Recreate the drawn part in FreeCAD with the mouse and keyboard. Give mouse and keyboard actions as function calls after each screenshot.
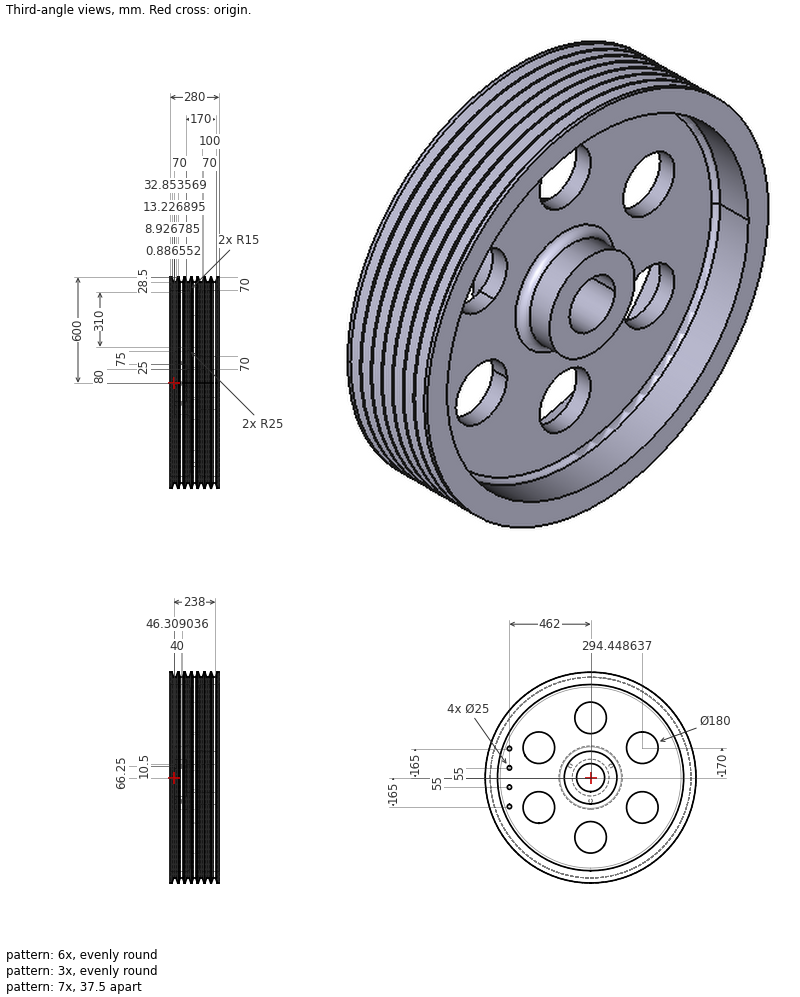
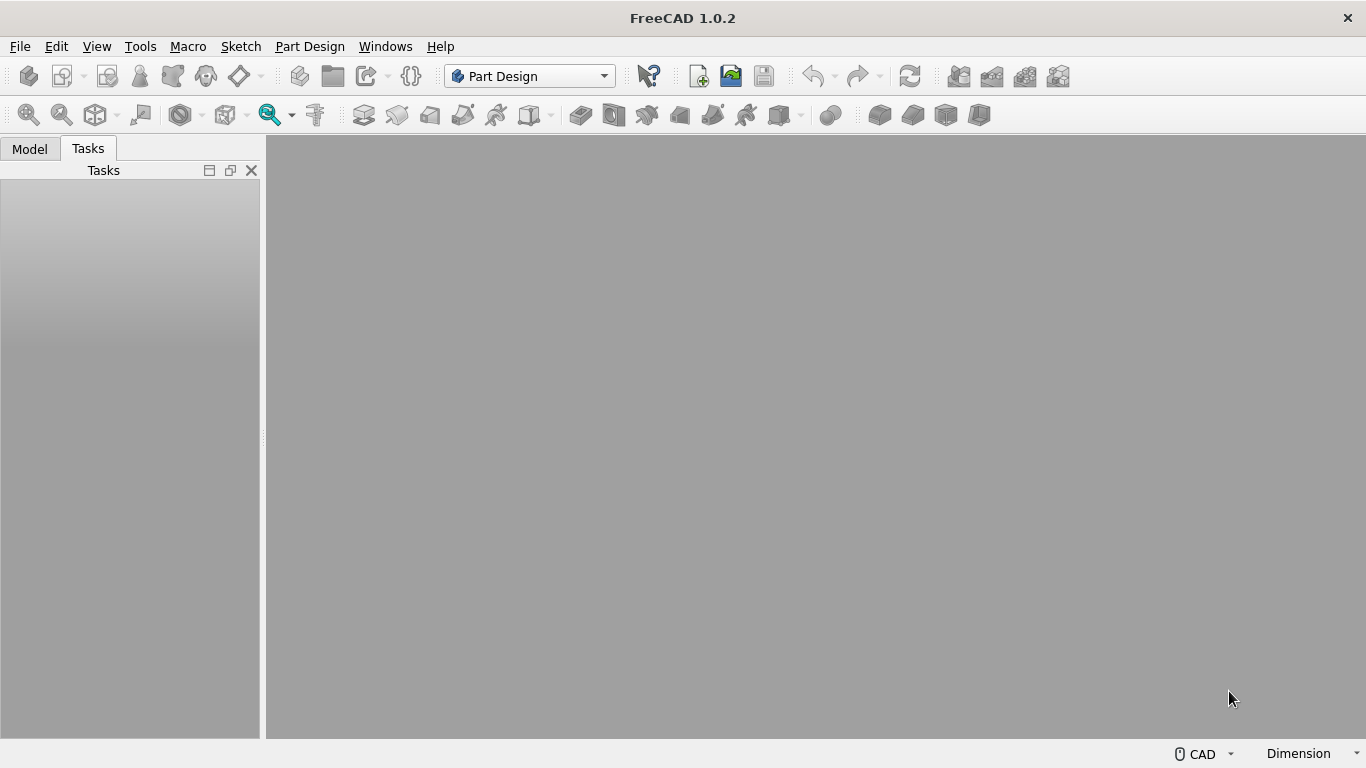
click(698, 76)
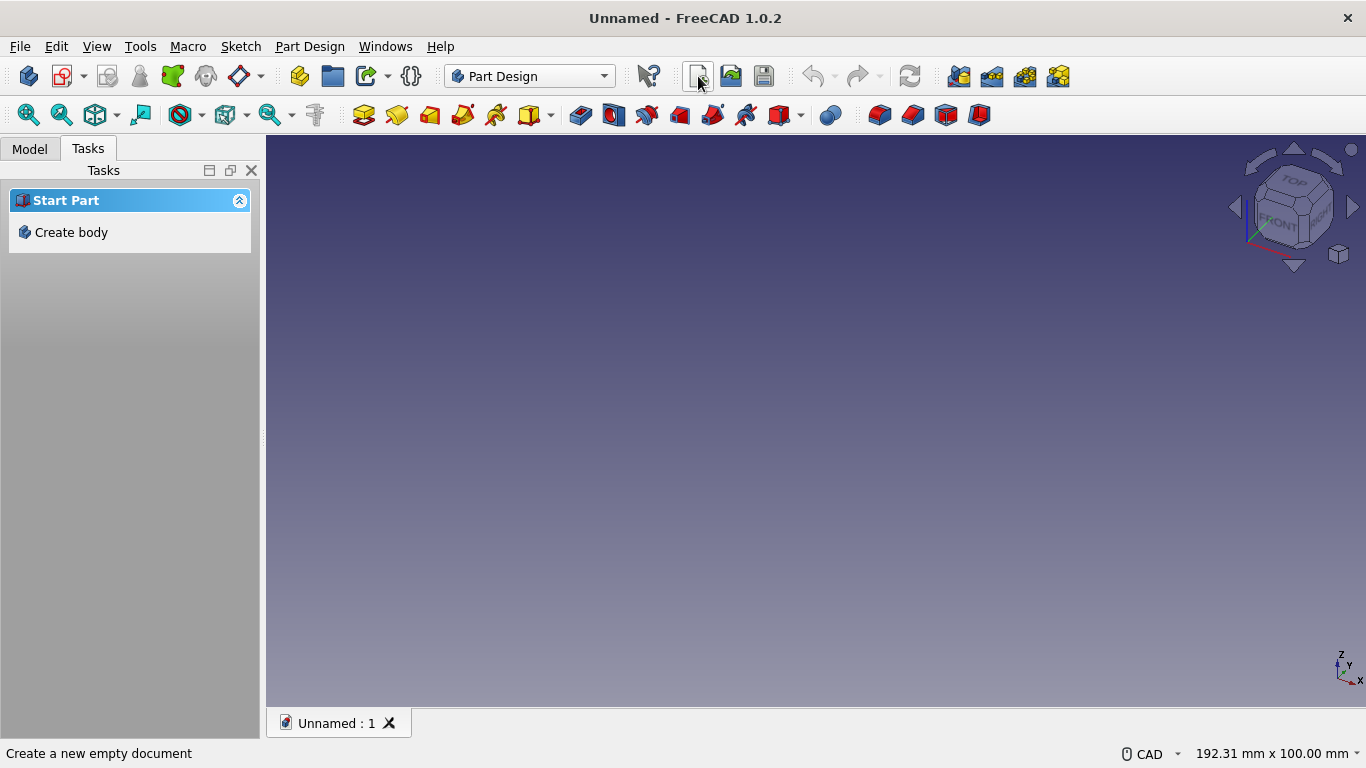
click(62, 76)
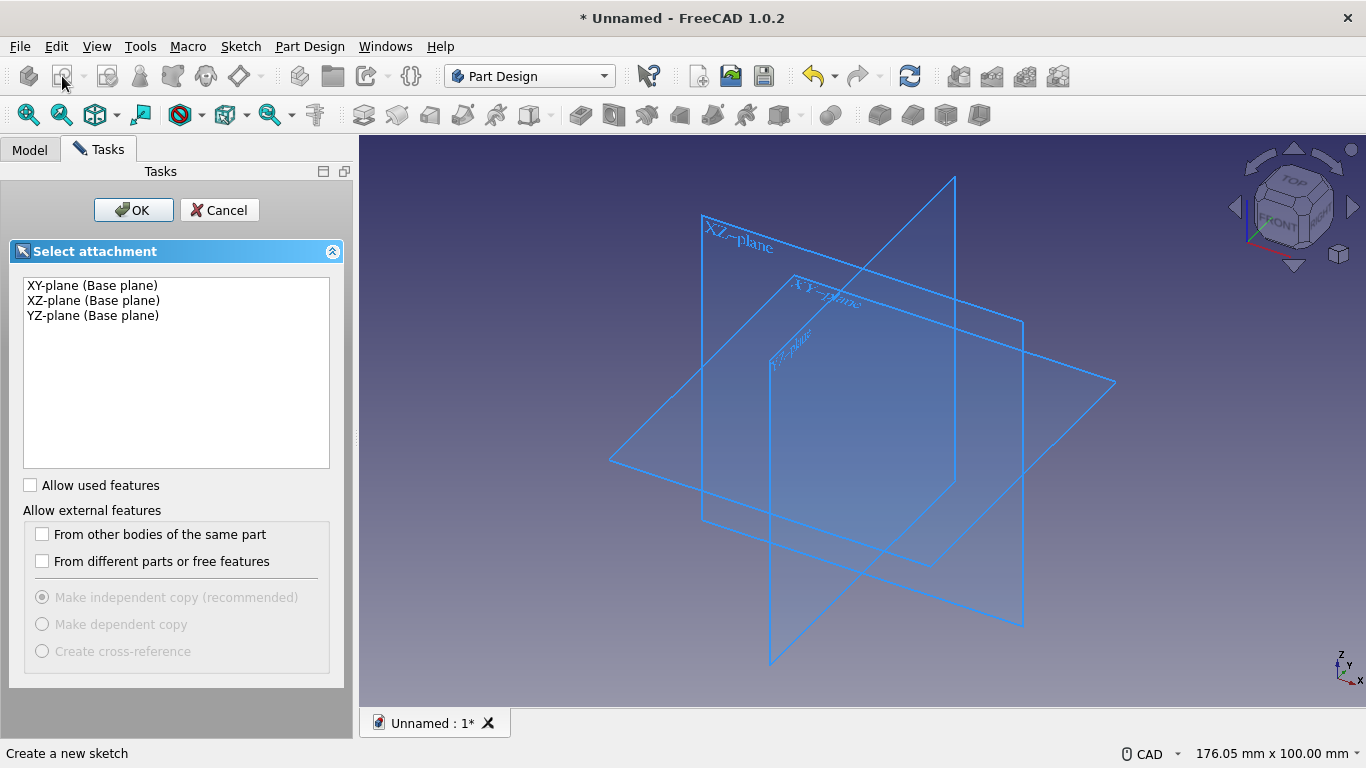
click(84, 286)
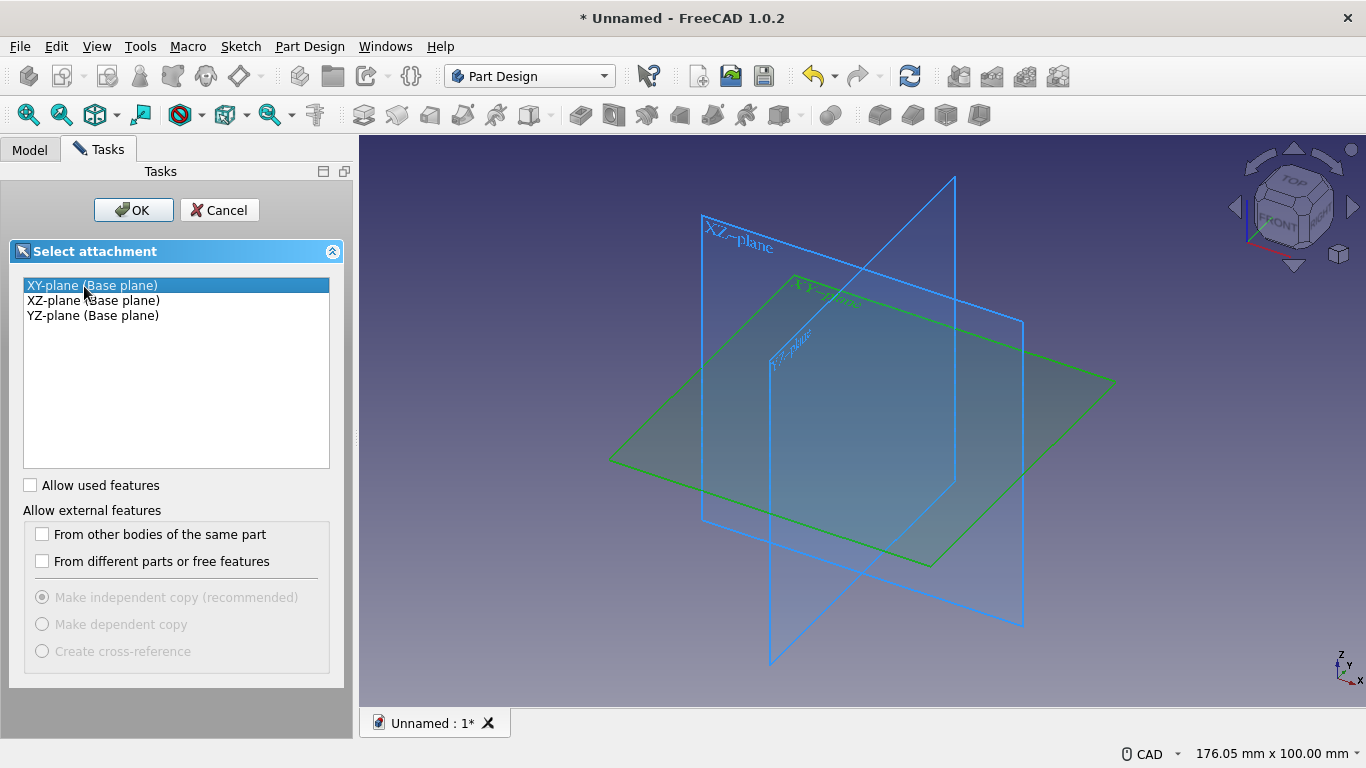
click(134, 210)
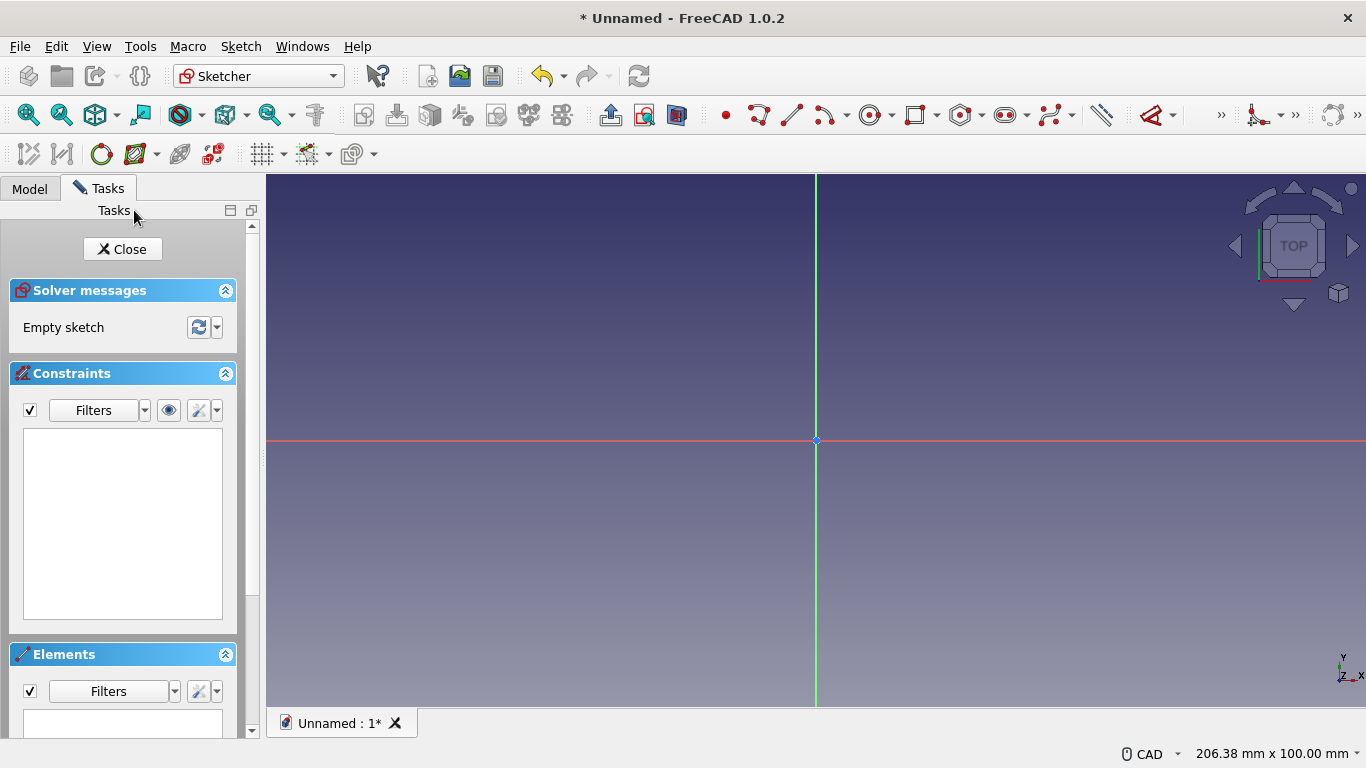
scroll(659, 640, down, 11)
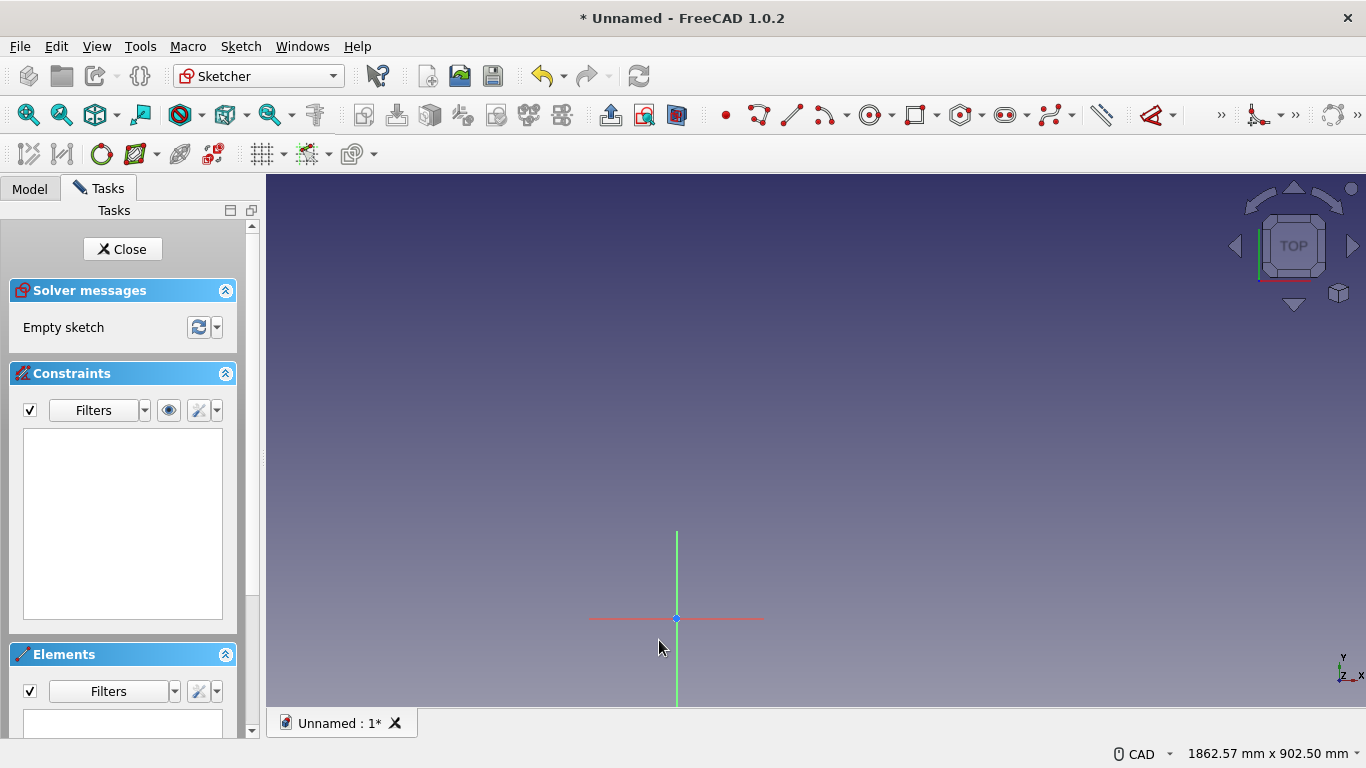
key(g)
key(l)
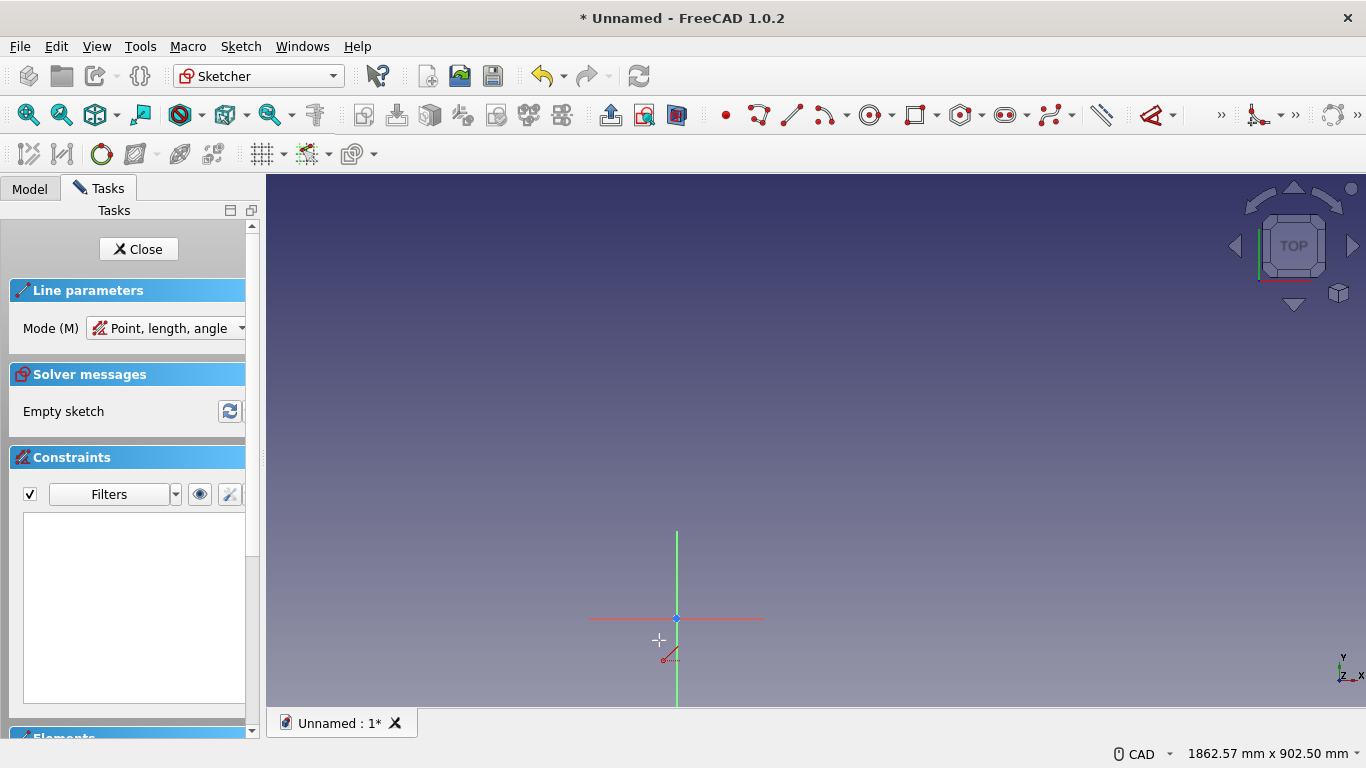
click(733, 315)
click(733, 498)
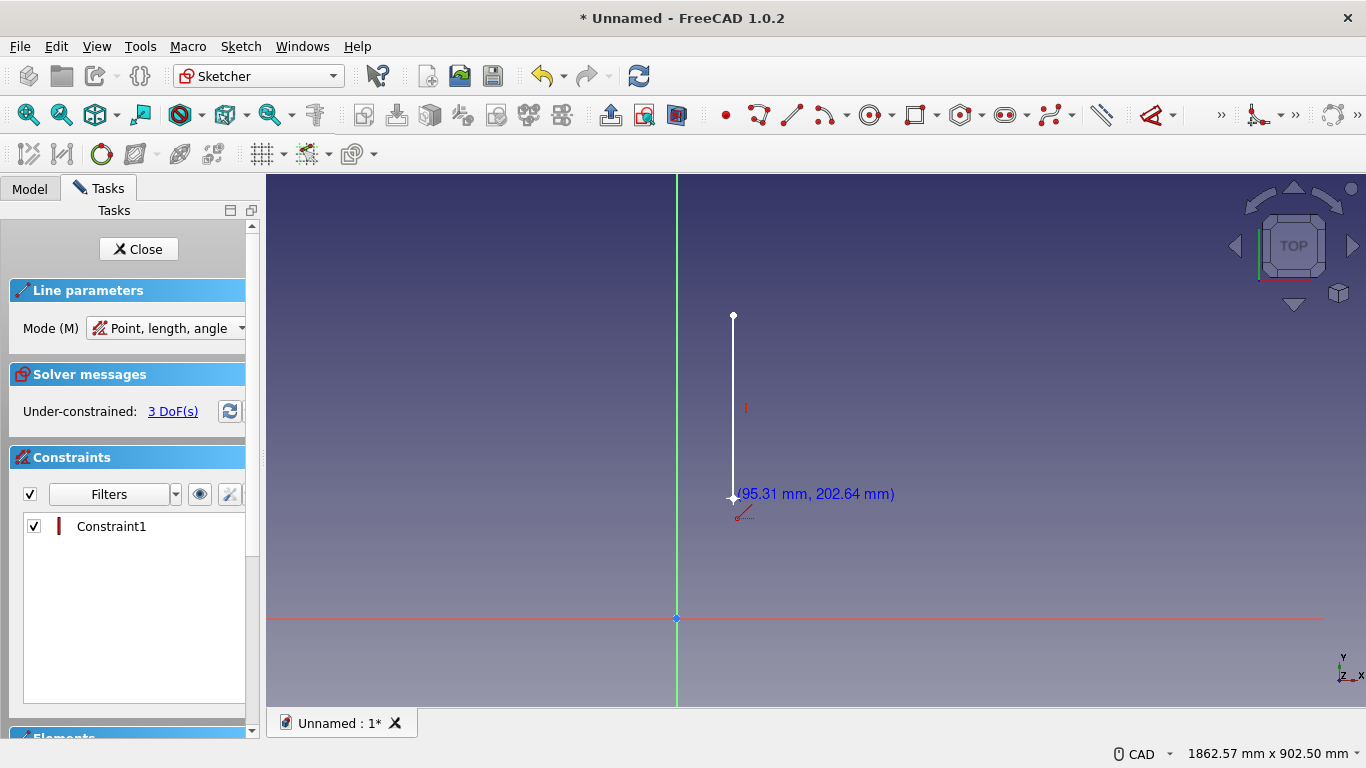
click(759, 116)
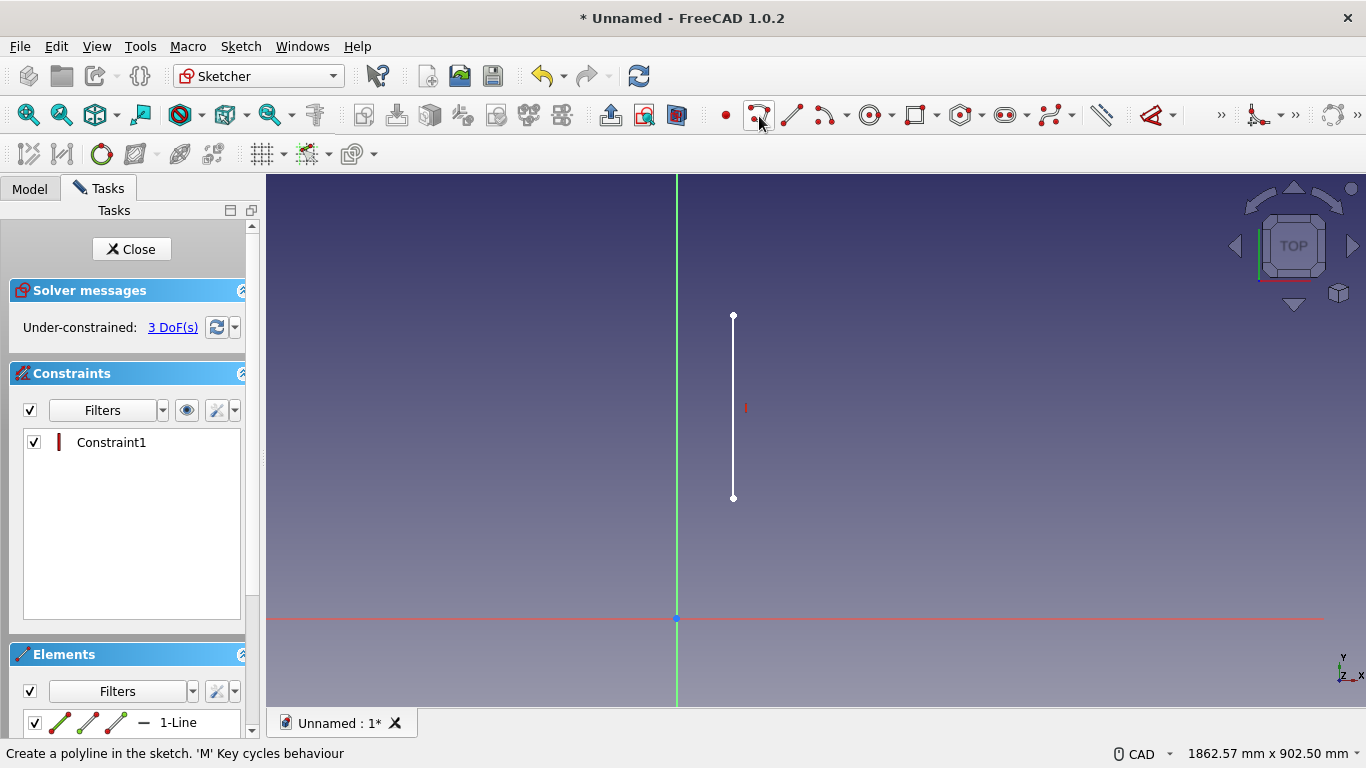
click(718, 512)
click(677, 512)
click(686, 557)
click(718, 557)
click(718, 571)
click(818, 571)
click(818, 530)
click(777, 530)
right_click(777, 530)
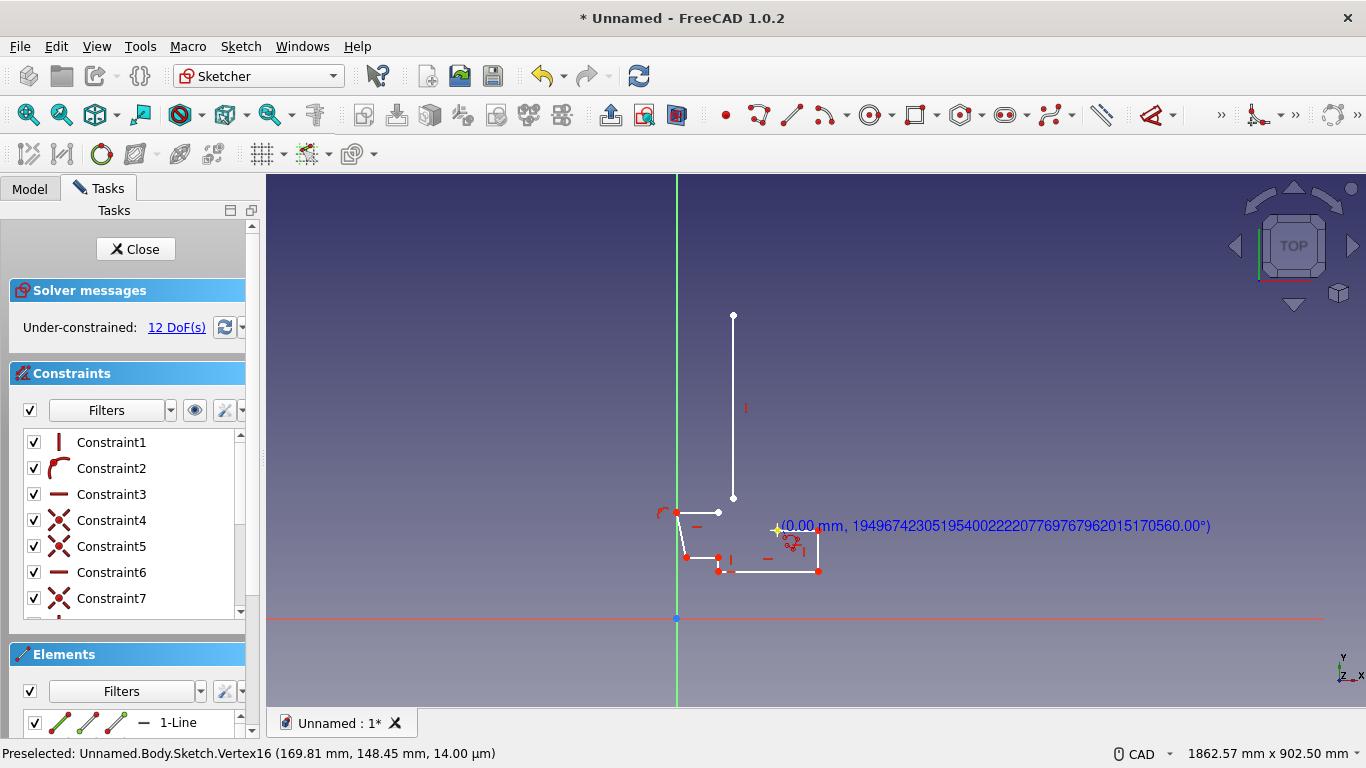
click(792, 116)